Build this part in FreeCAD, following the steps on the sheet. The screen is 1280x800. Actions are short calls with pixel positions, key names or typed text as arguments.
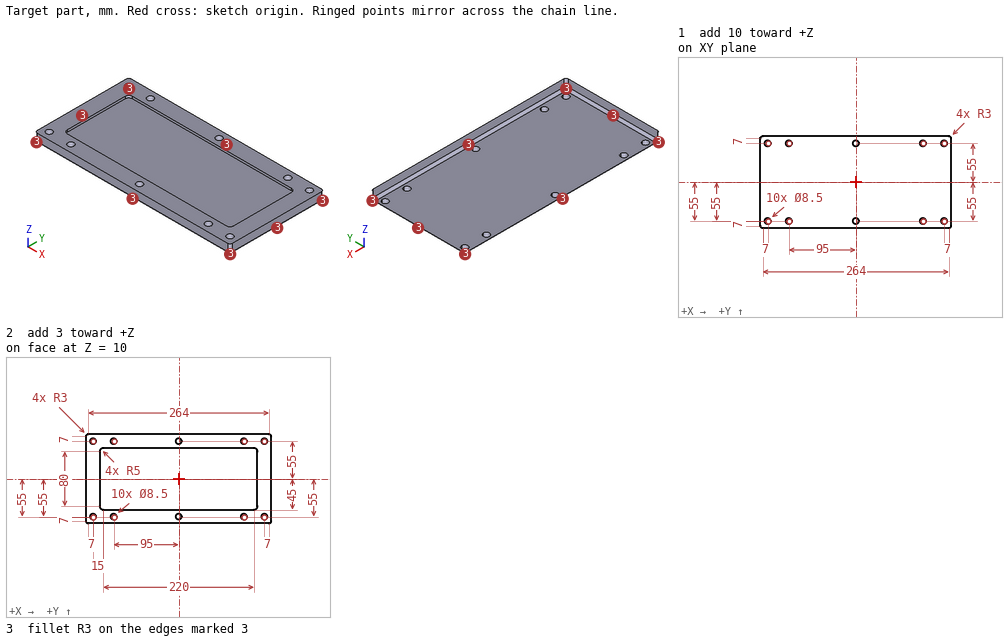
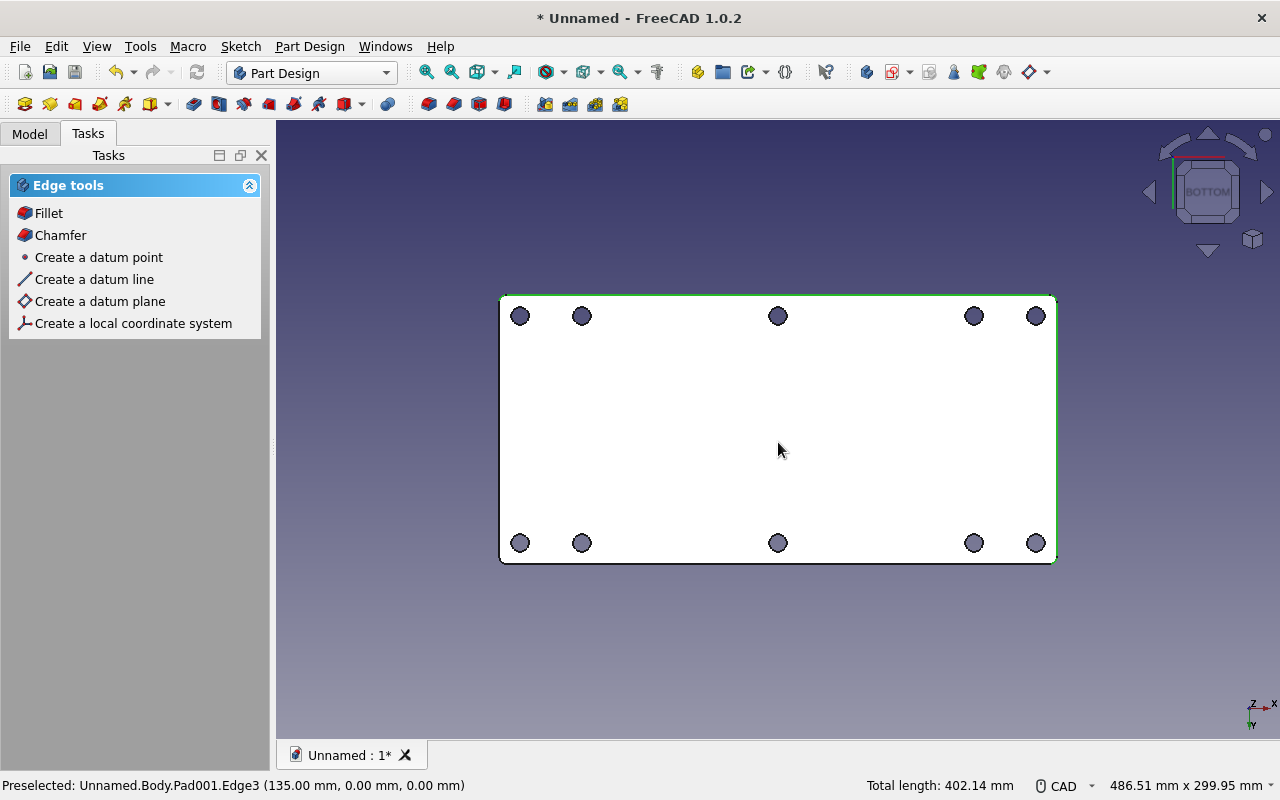
click(778, 563, ctrl)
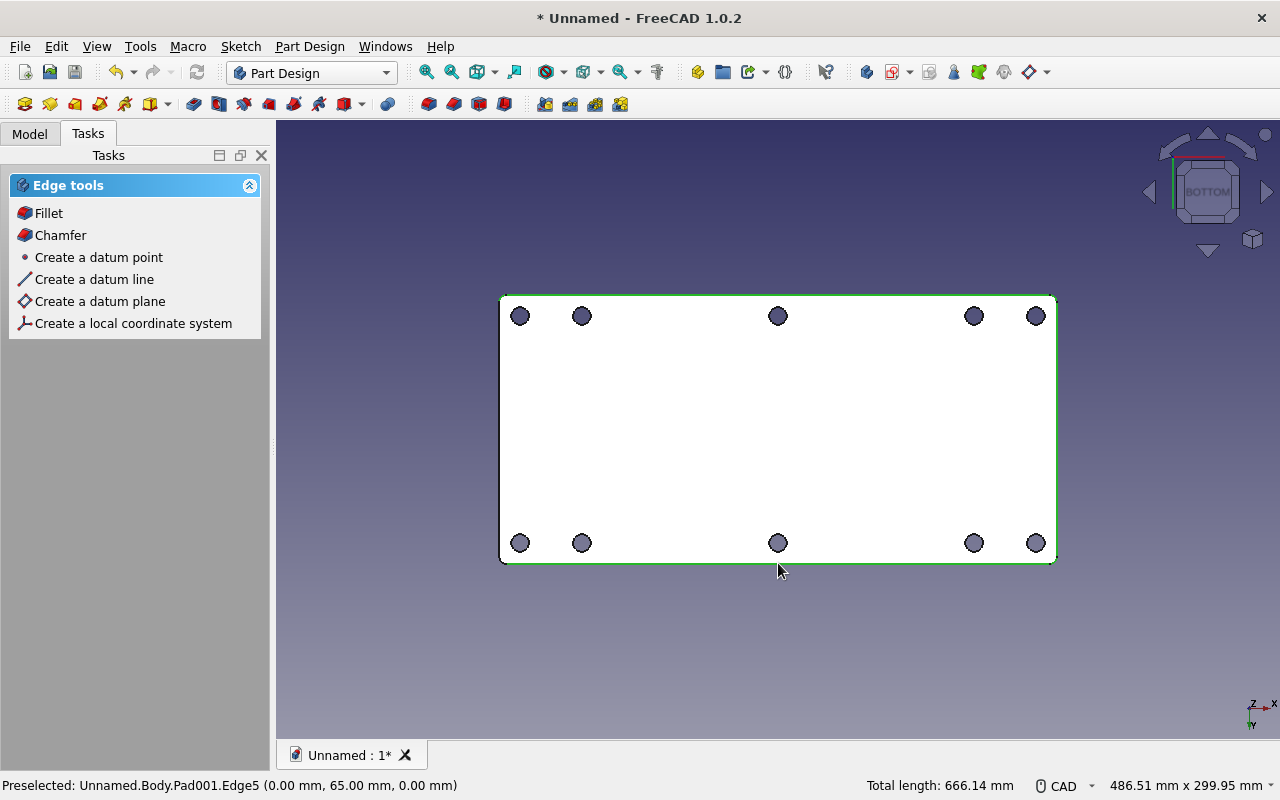
click(499, 428, ctrl)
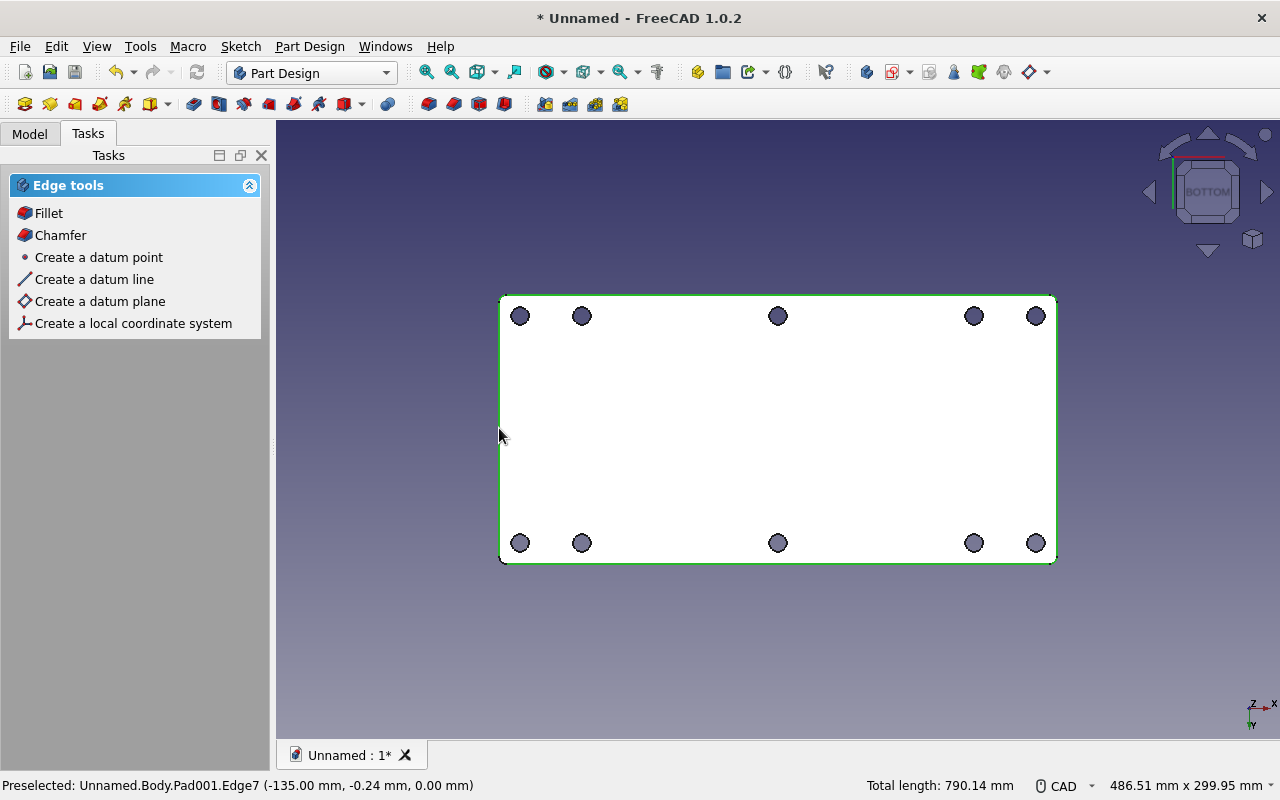
scroll(501, 561, up, 8)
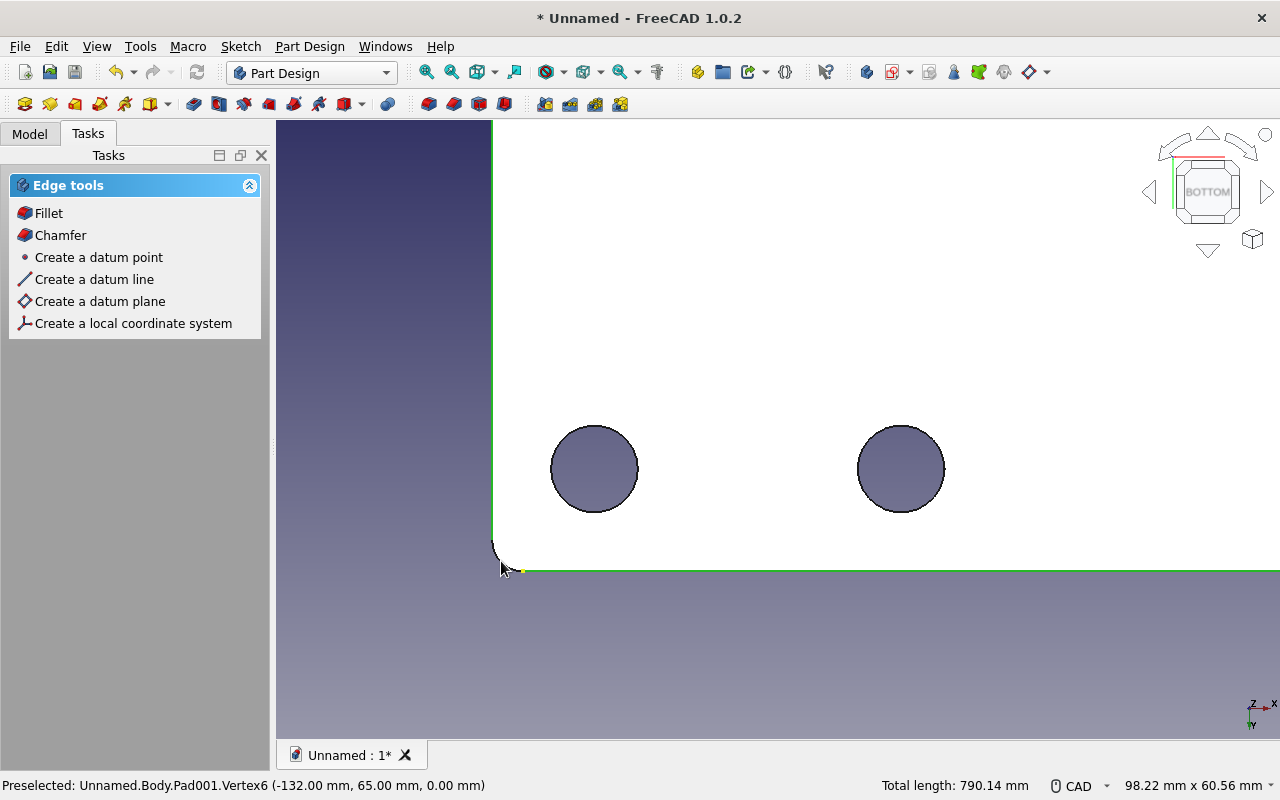
click(501, 561, ctrl)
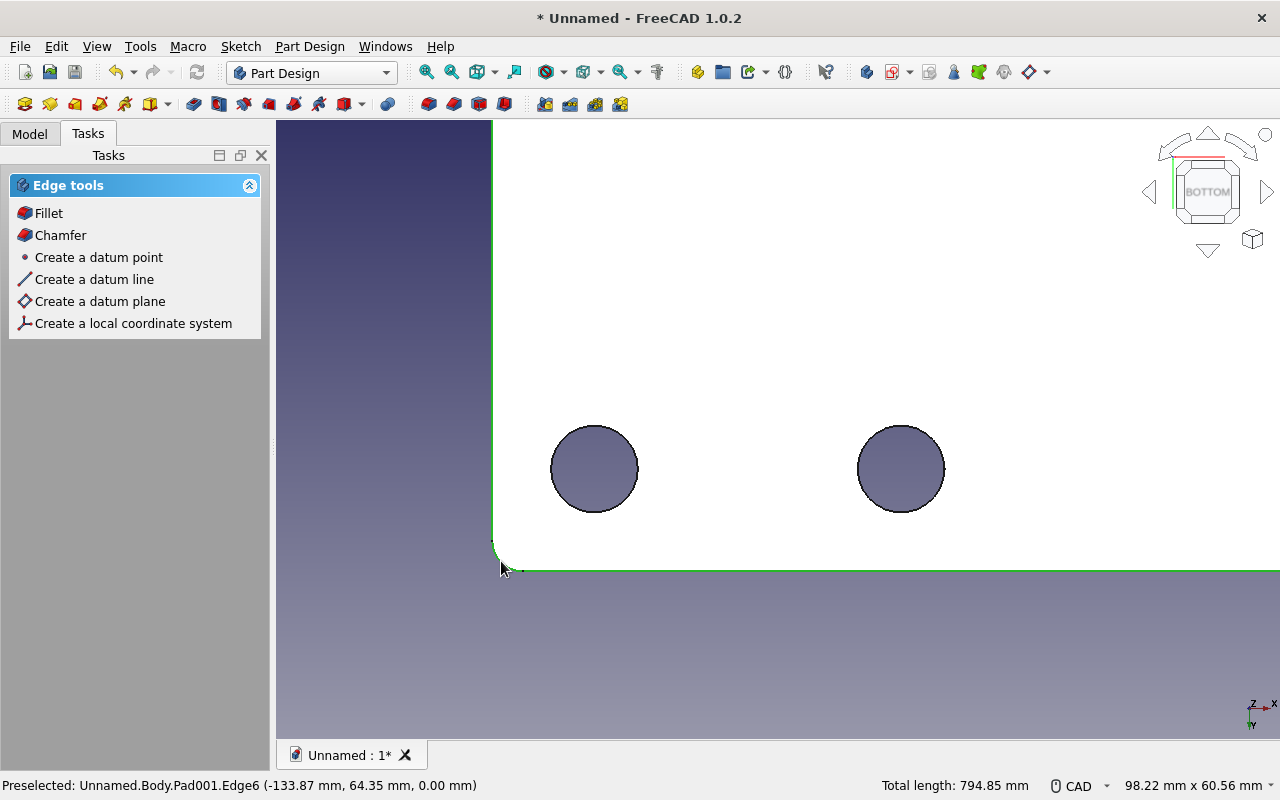
click(429, 104)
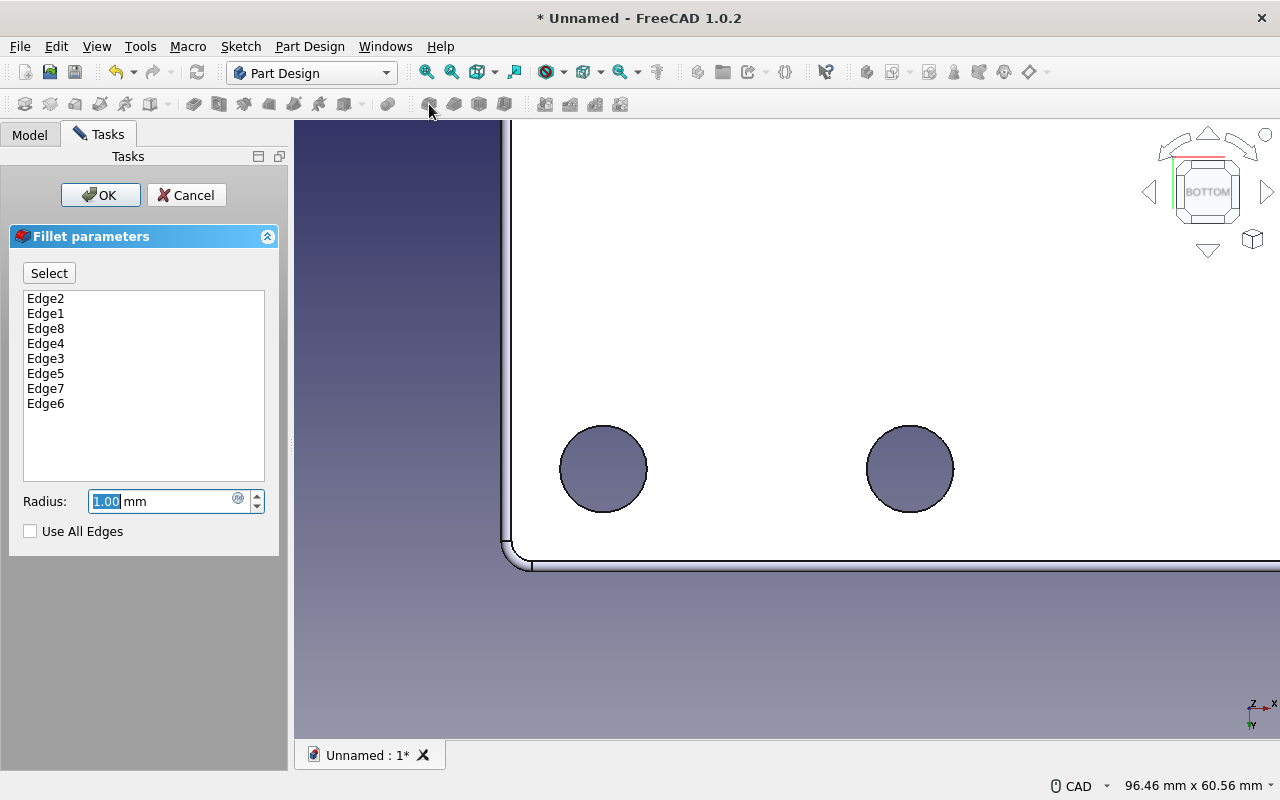
text(3)
key(Tab)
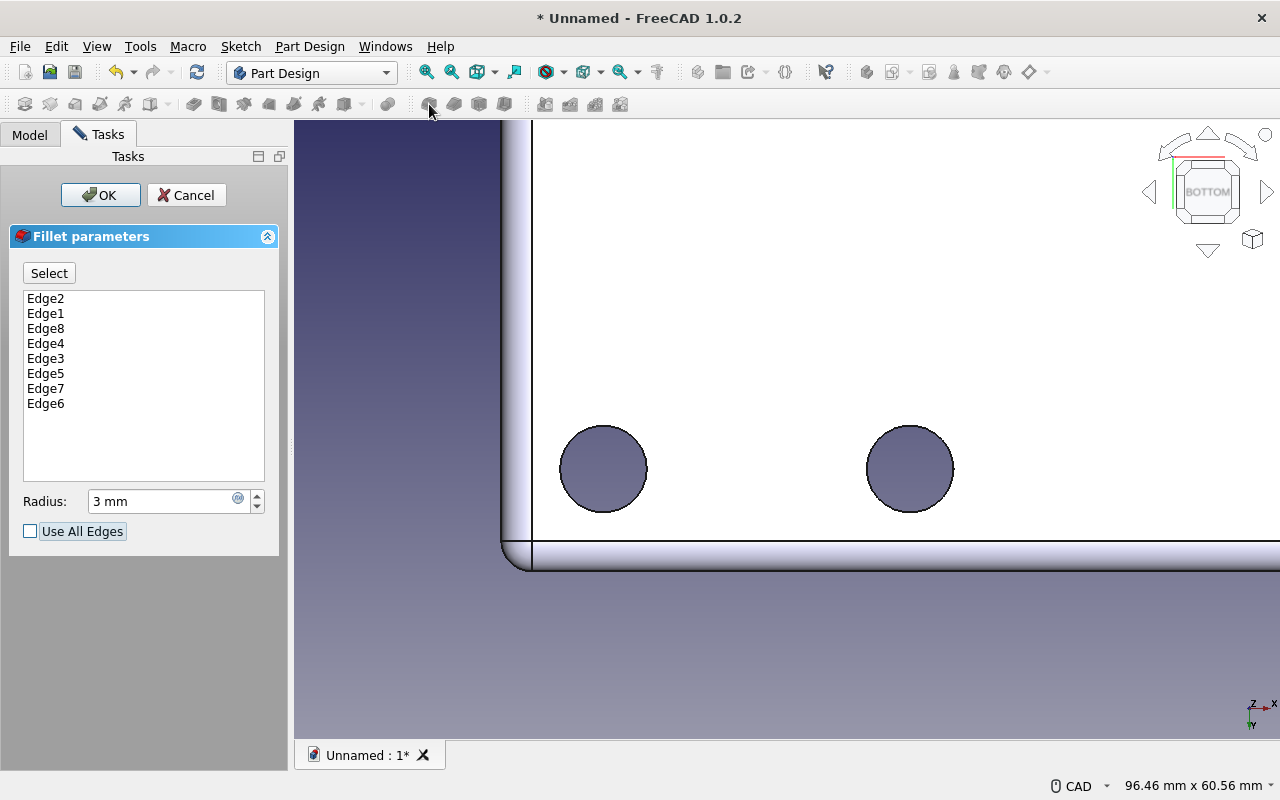
click(101, 195)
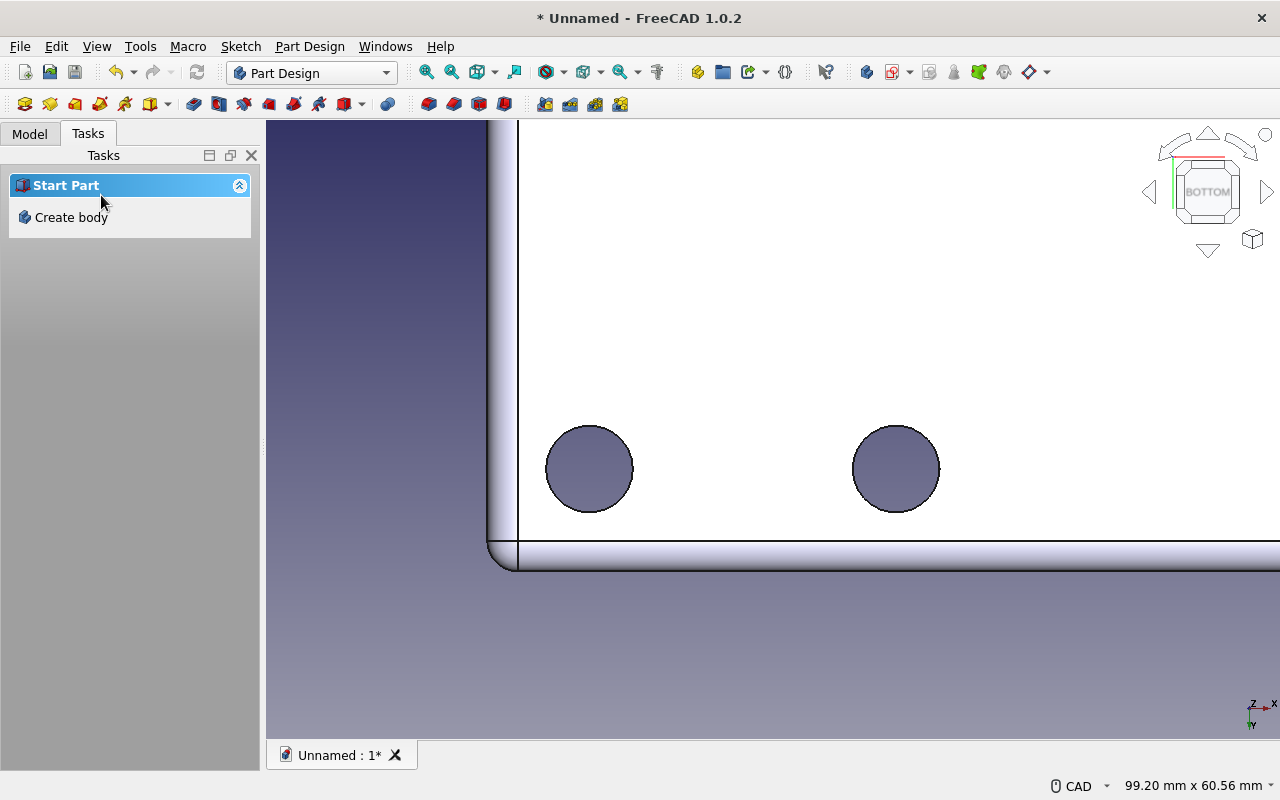
key(0)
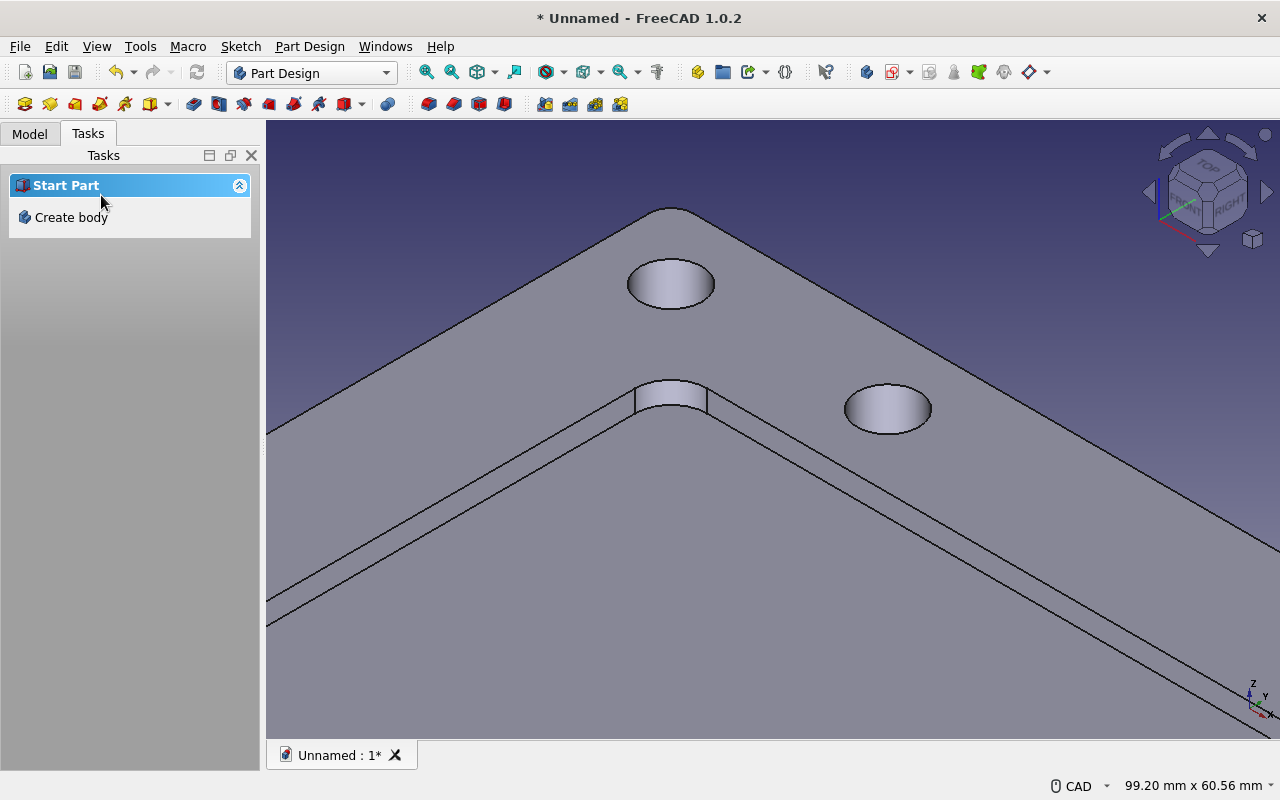
click(427, 72)